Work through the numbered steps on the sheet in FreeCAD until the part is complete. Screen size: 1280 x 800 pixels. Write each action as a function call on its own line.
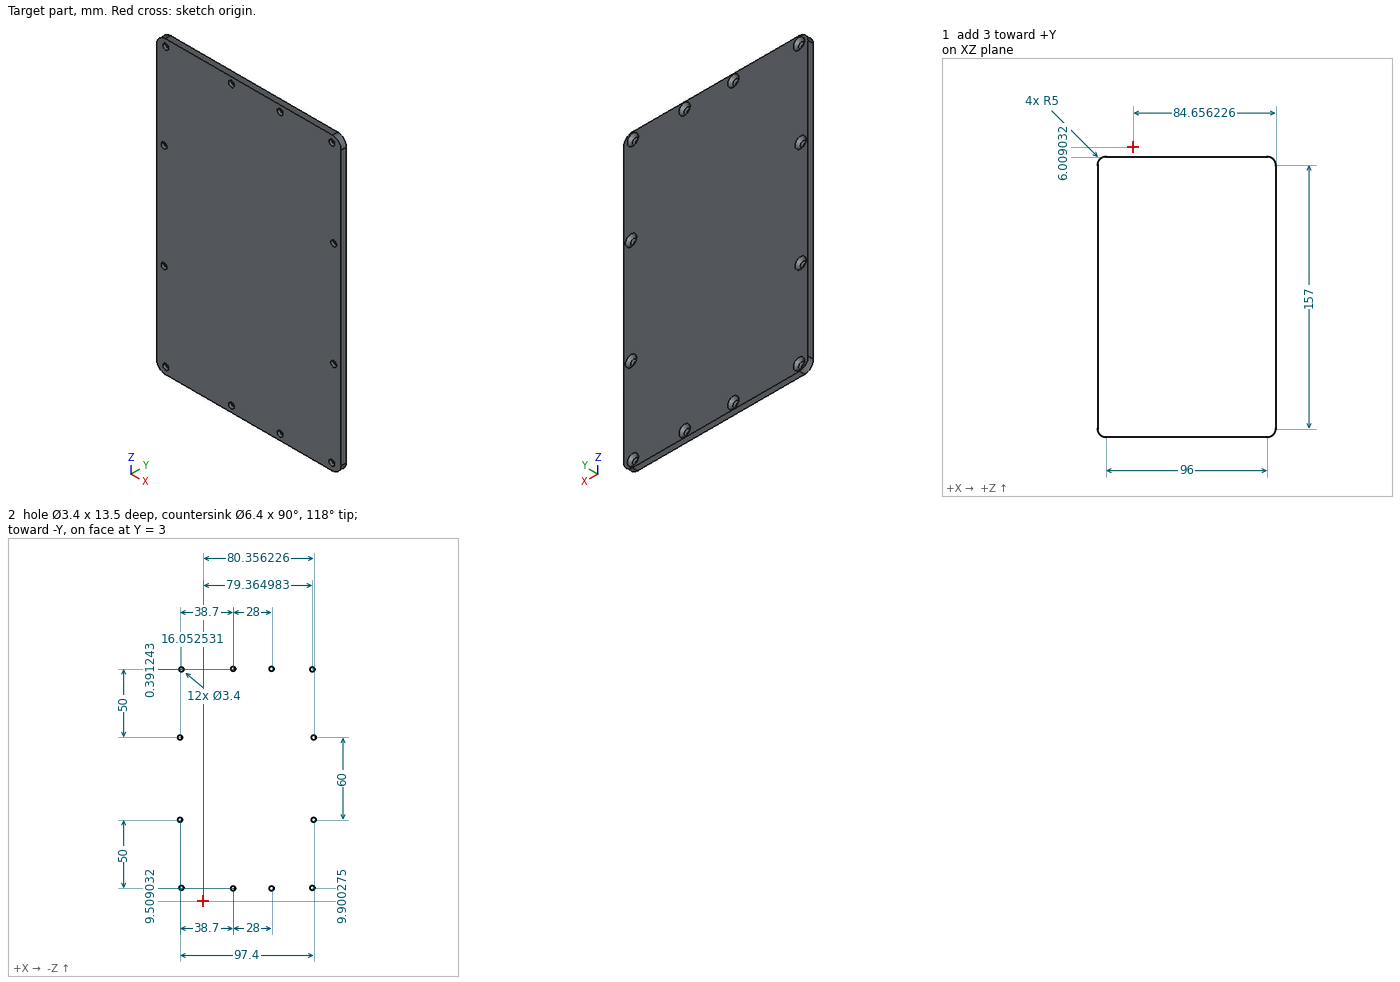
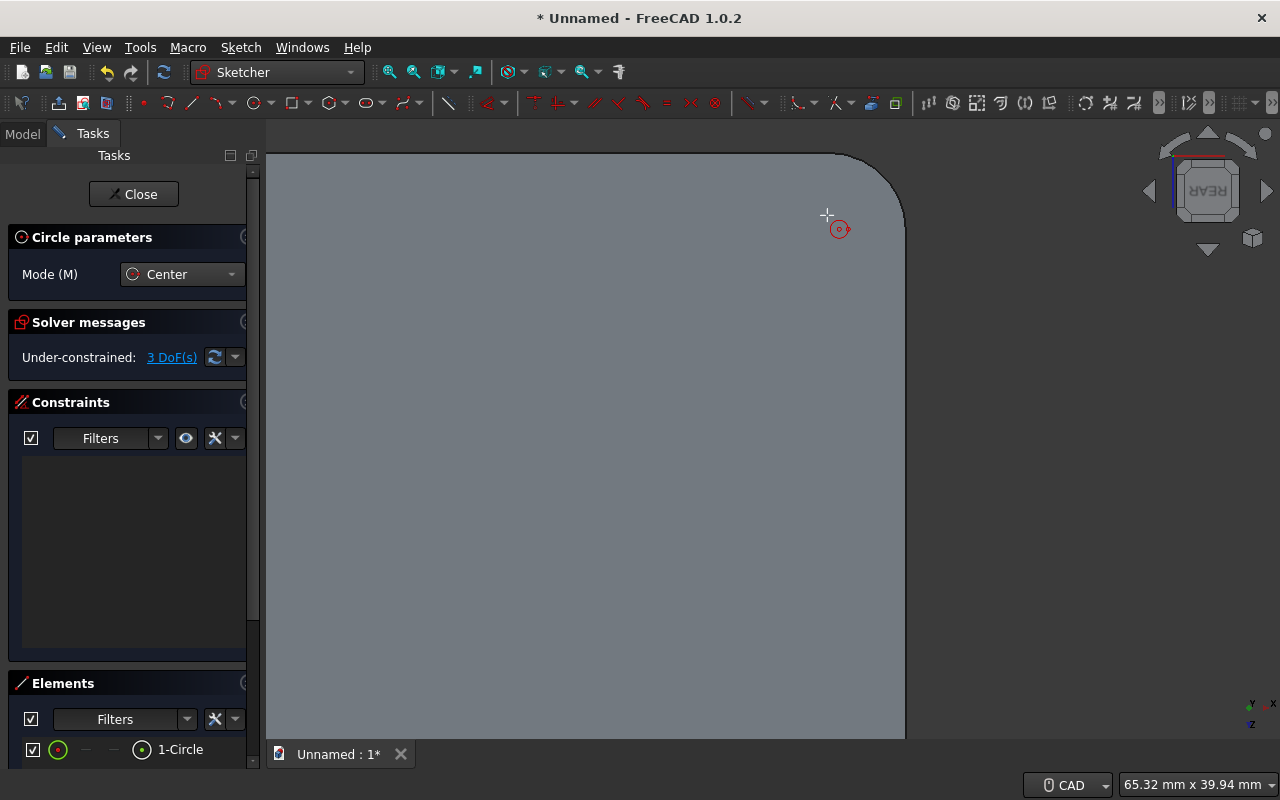
scroll(828, 215, down, 9)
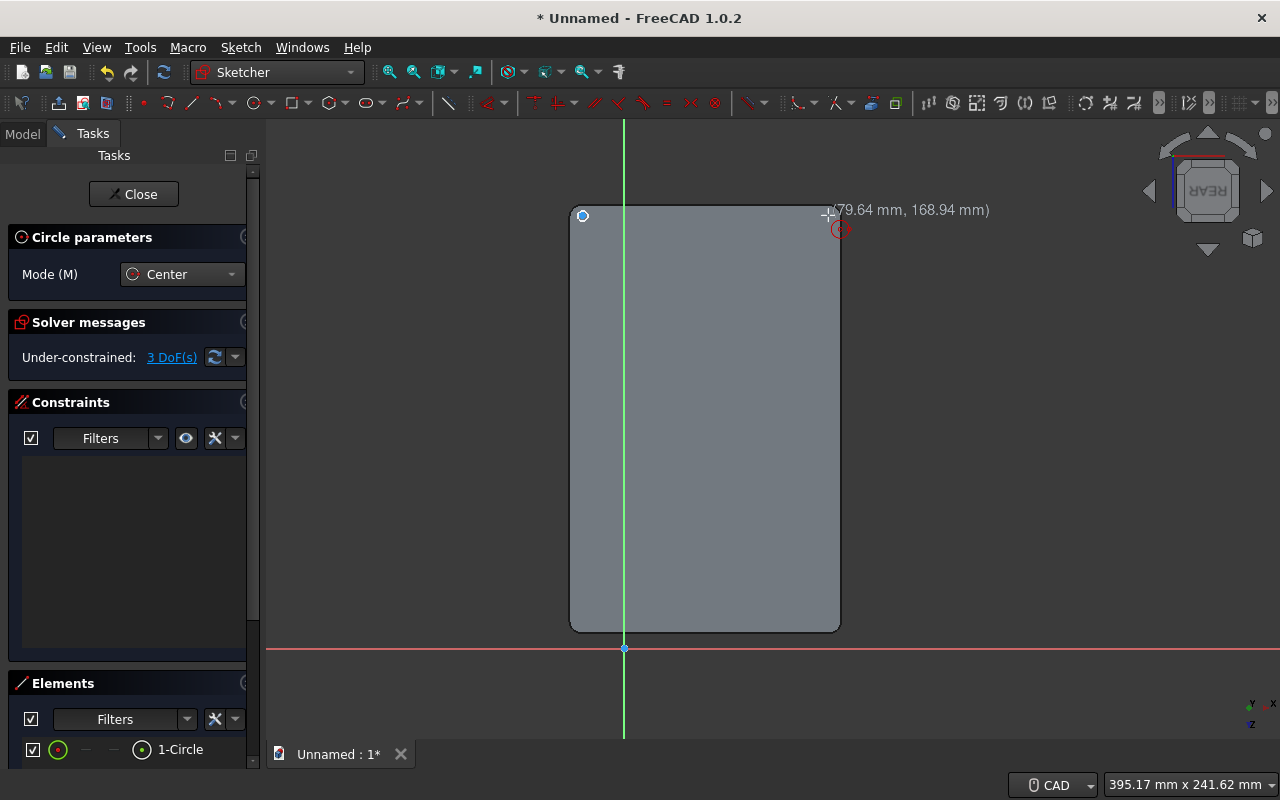
click(828, 215)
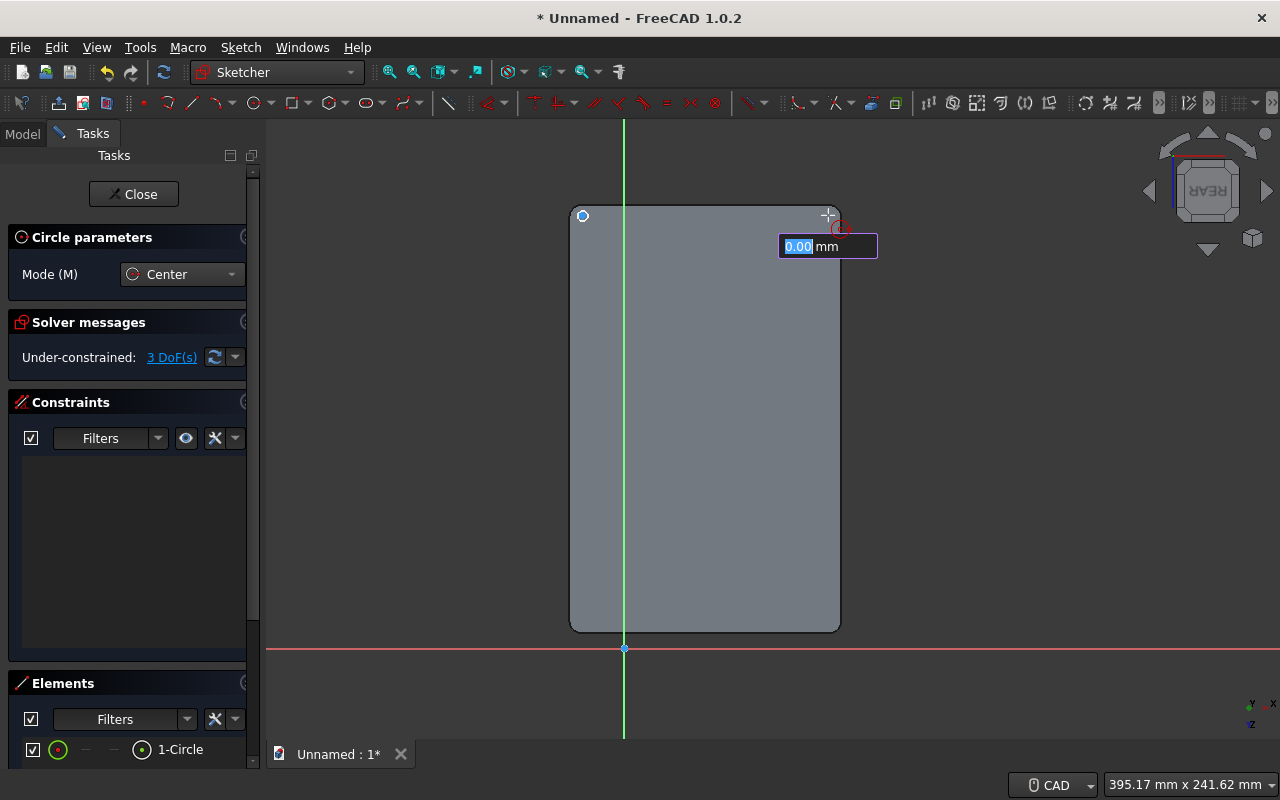
scroll(831, 212, up, 7)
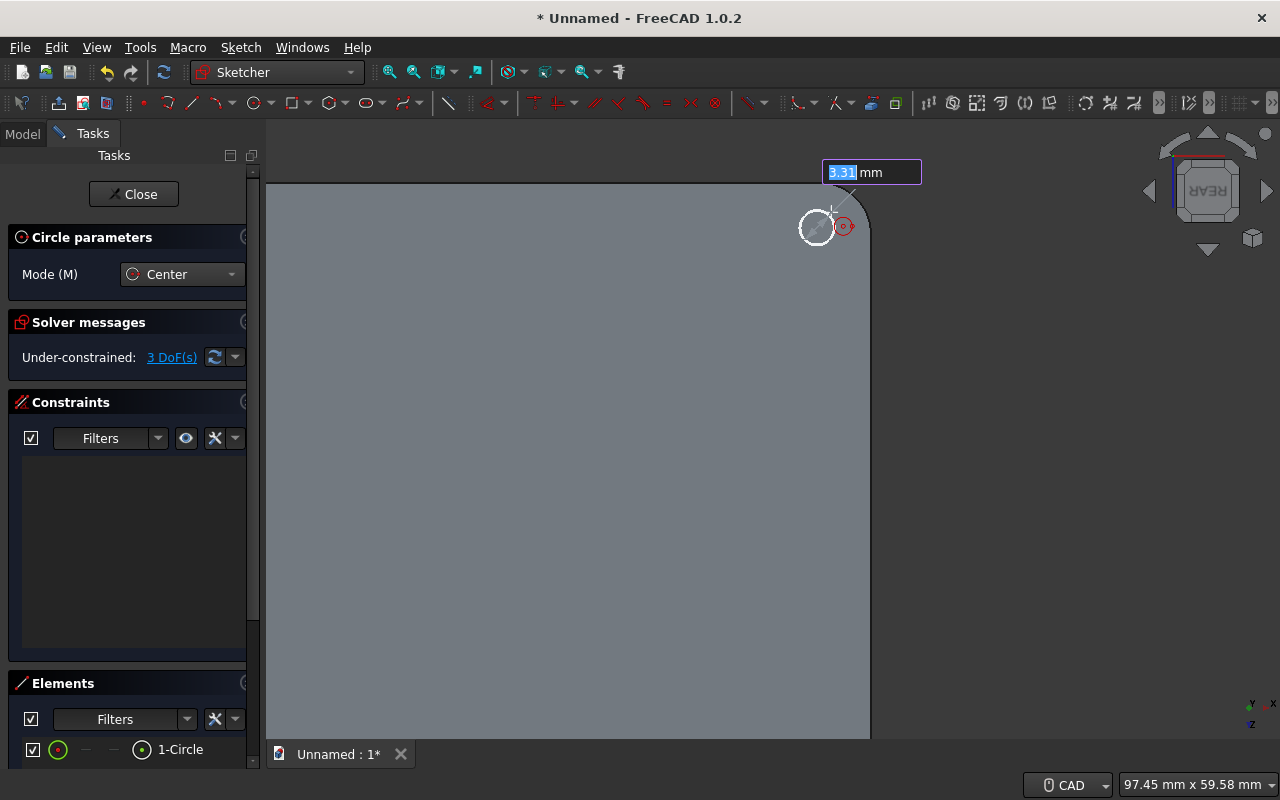
click(829, 211)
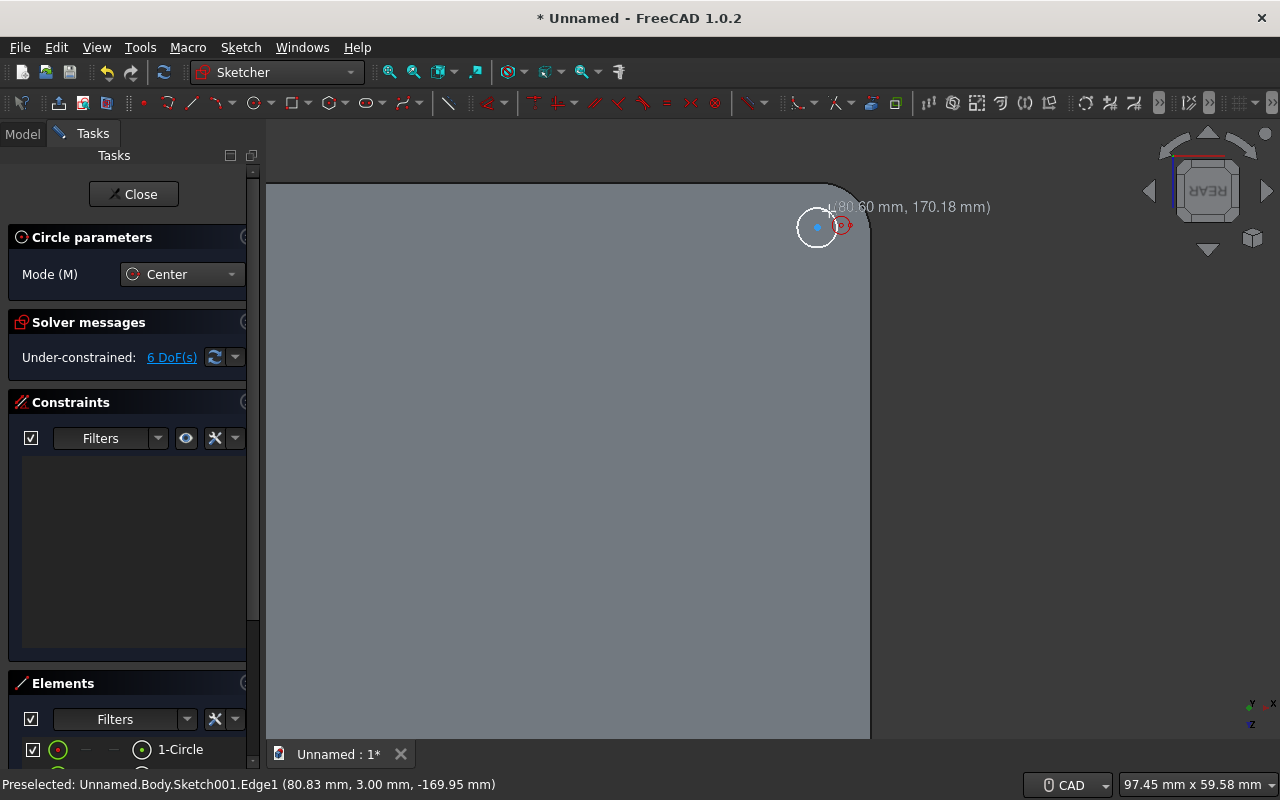
scroll(830, 212, down, 7)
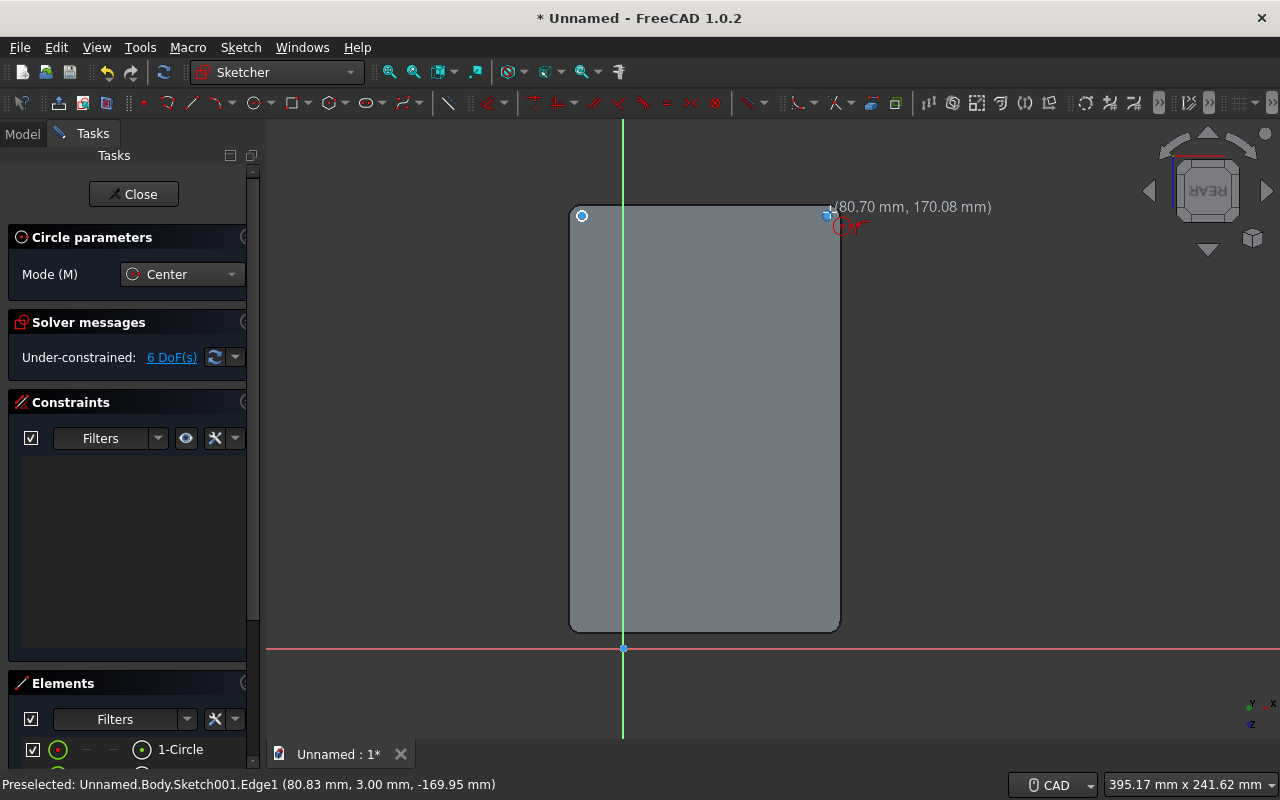
scroll(830, 342, up, 9)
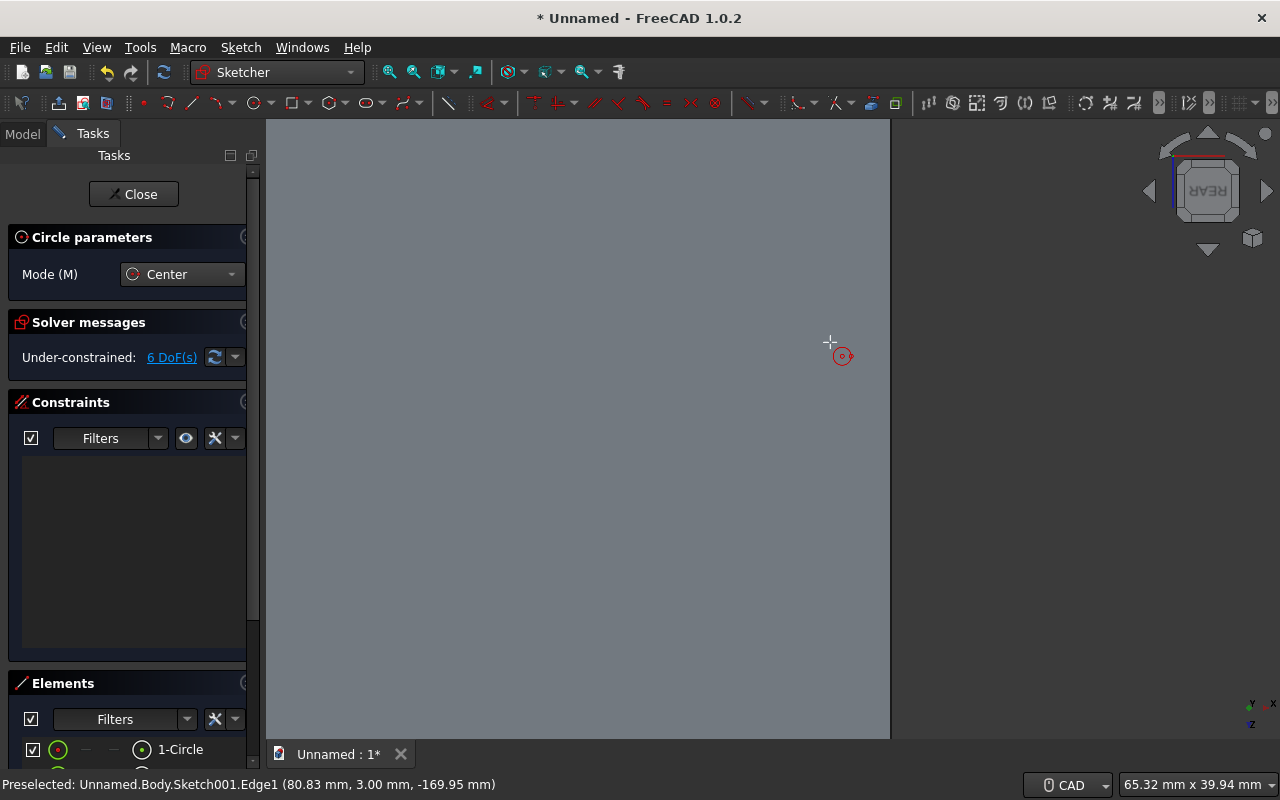
scroll(830, 342, down, 9)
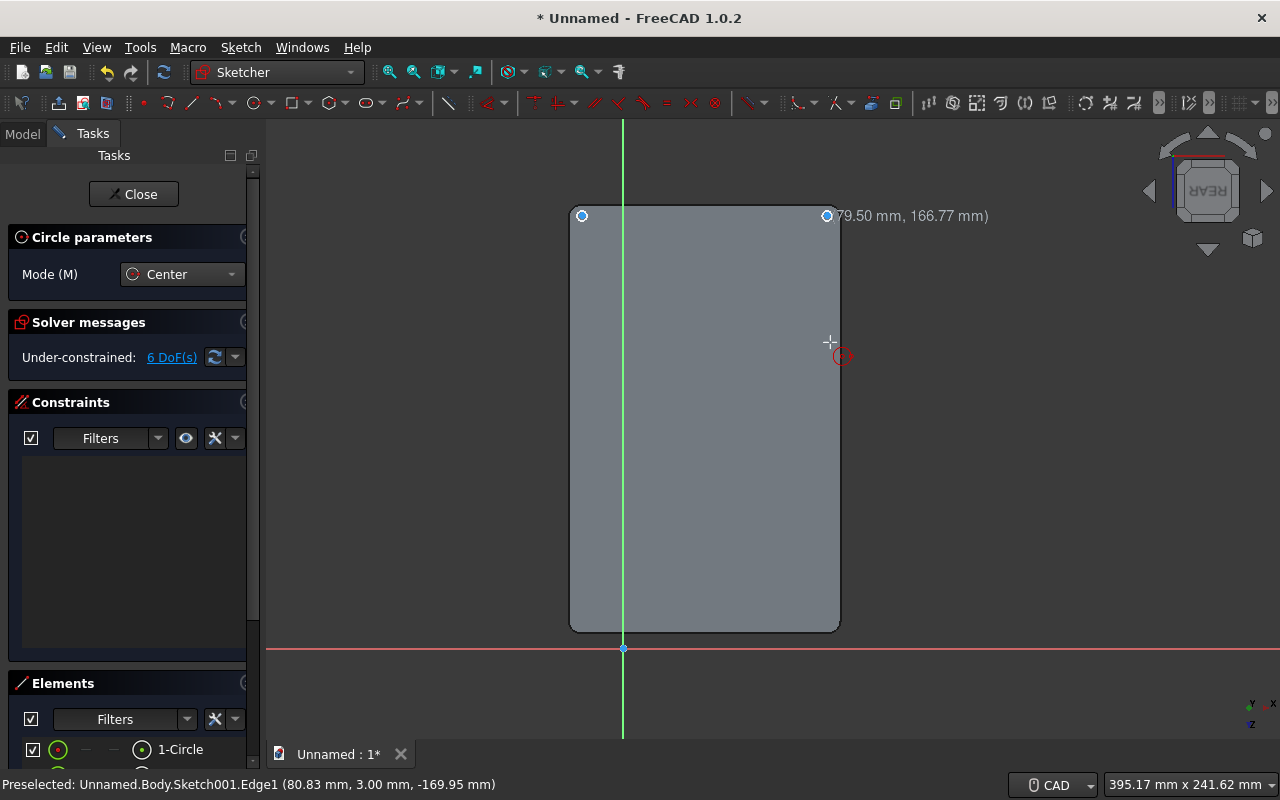
click(830, 342)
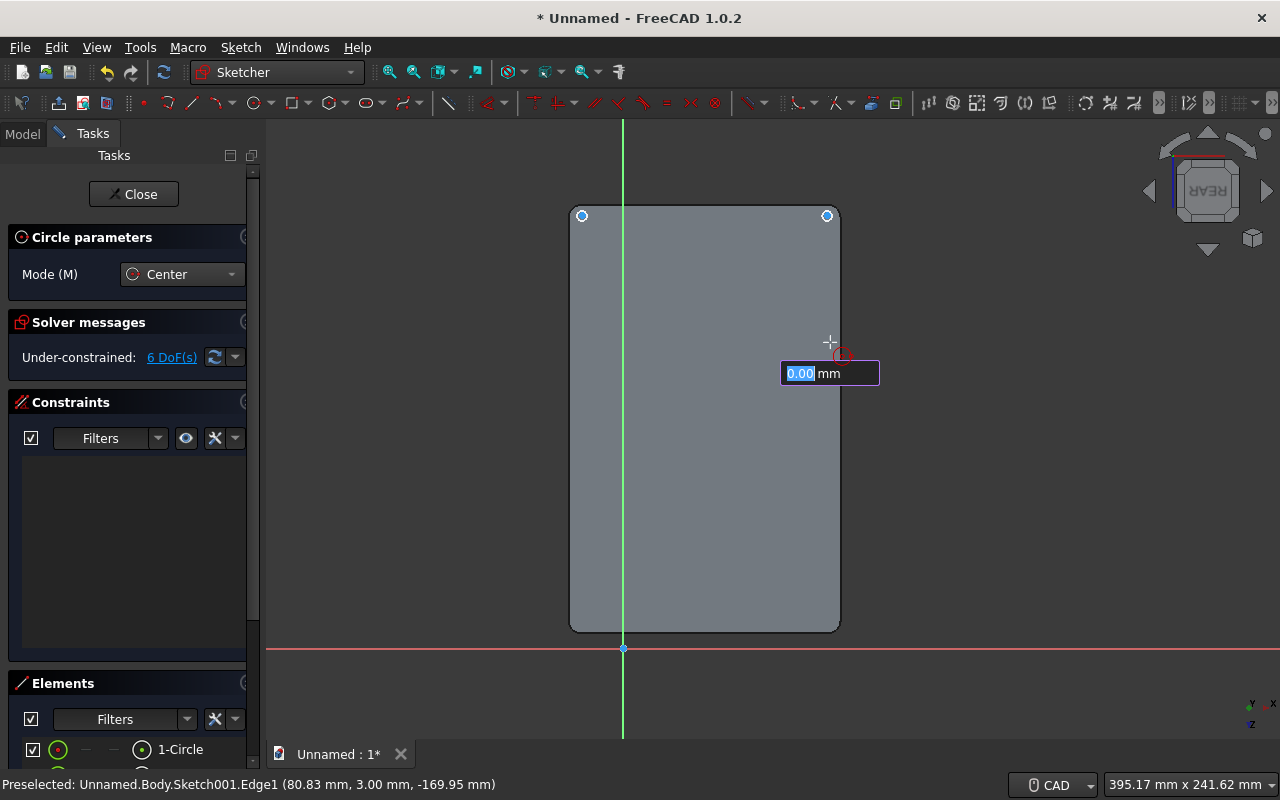
scroll(833, 339, up, 7)